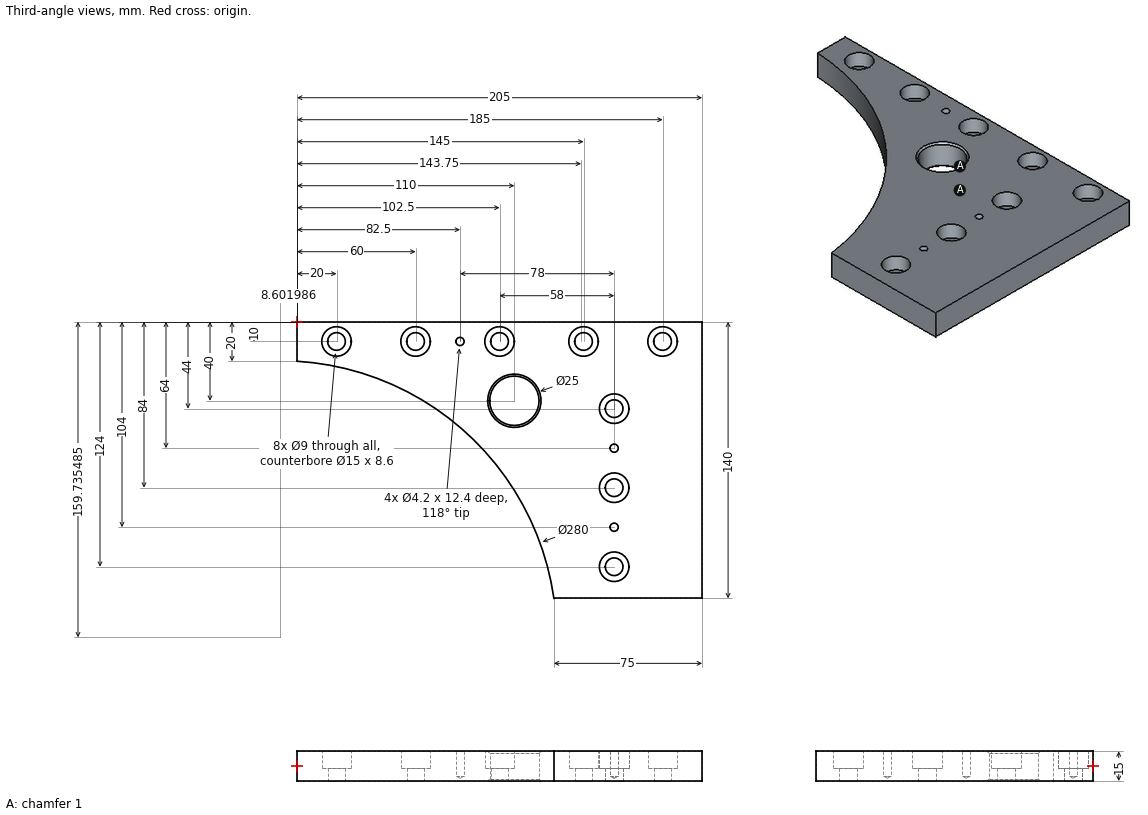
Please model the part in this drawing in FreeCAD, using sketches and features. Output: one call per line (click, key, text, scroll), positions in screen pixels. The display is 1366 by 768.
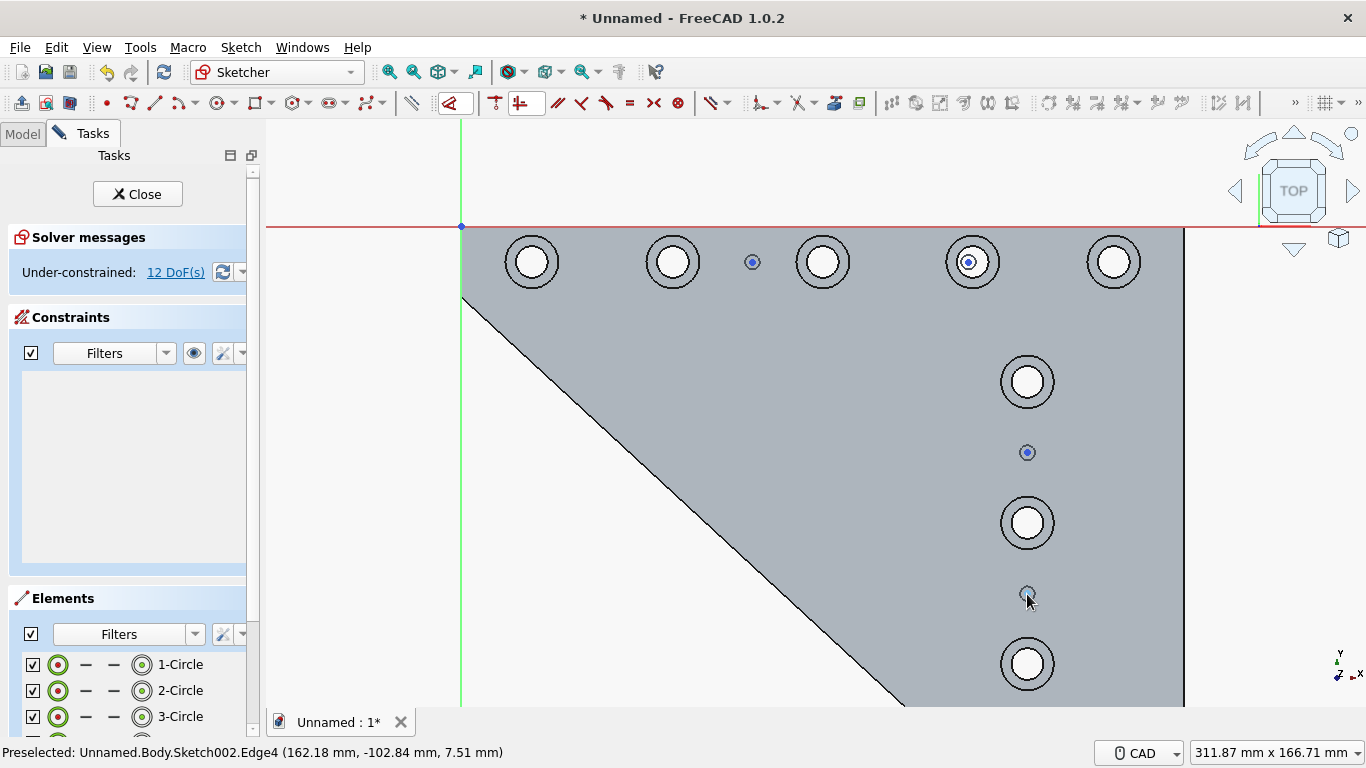
scroll(758, 257, up, 4)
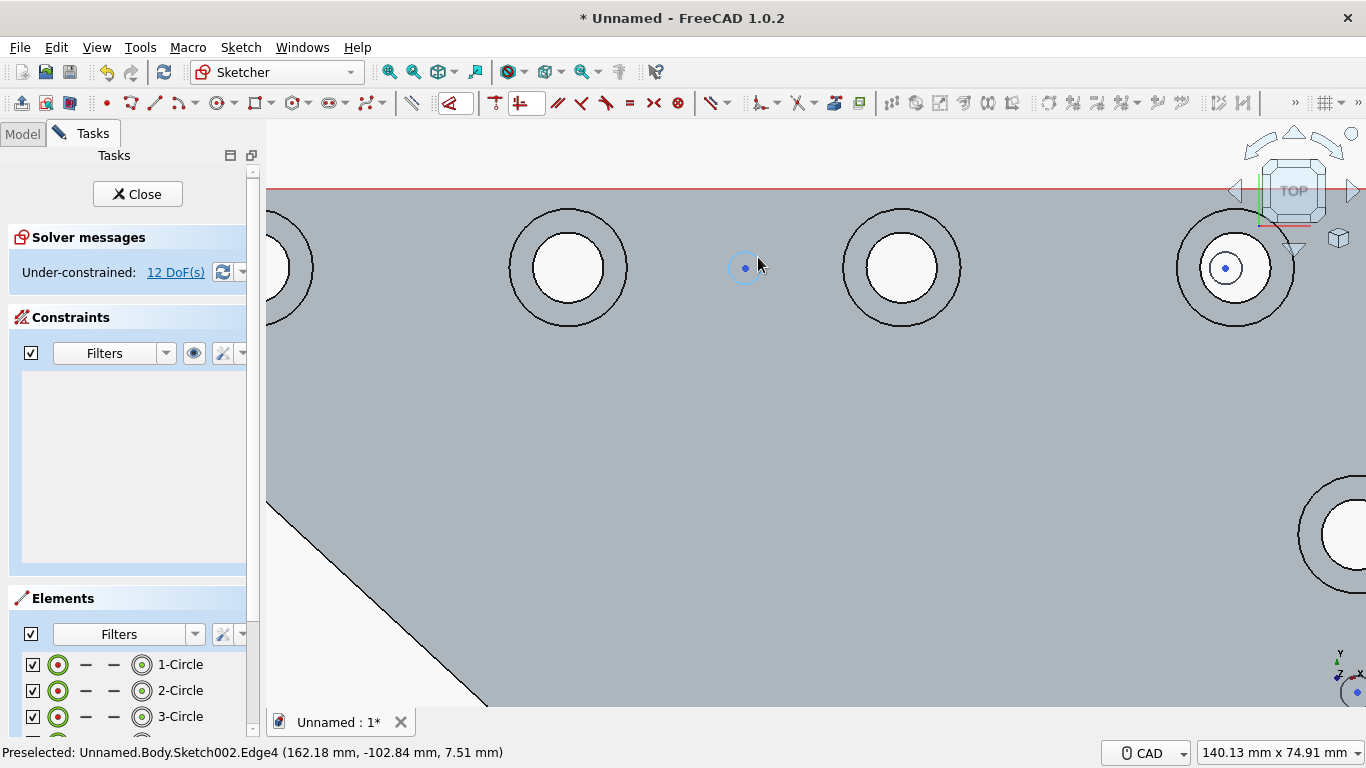
click(756, 257)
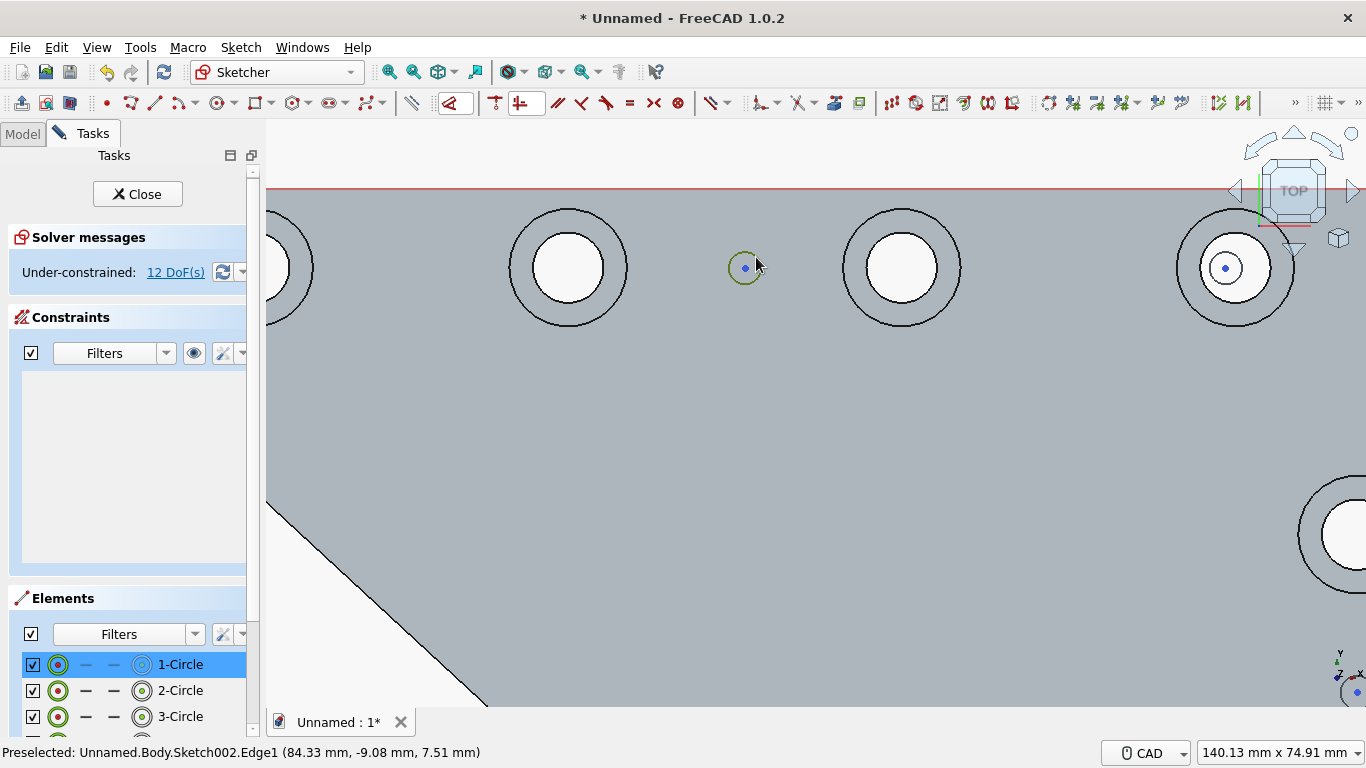
scroll(757, 256, down, 4)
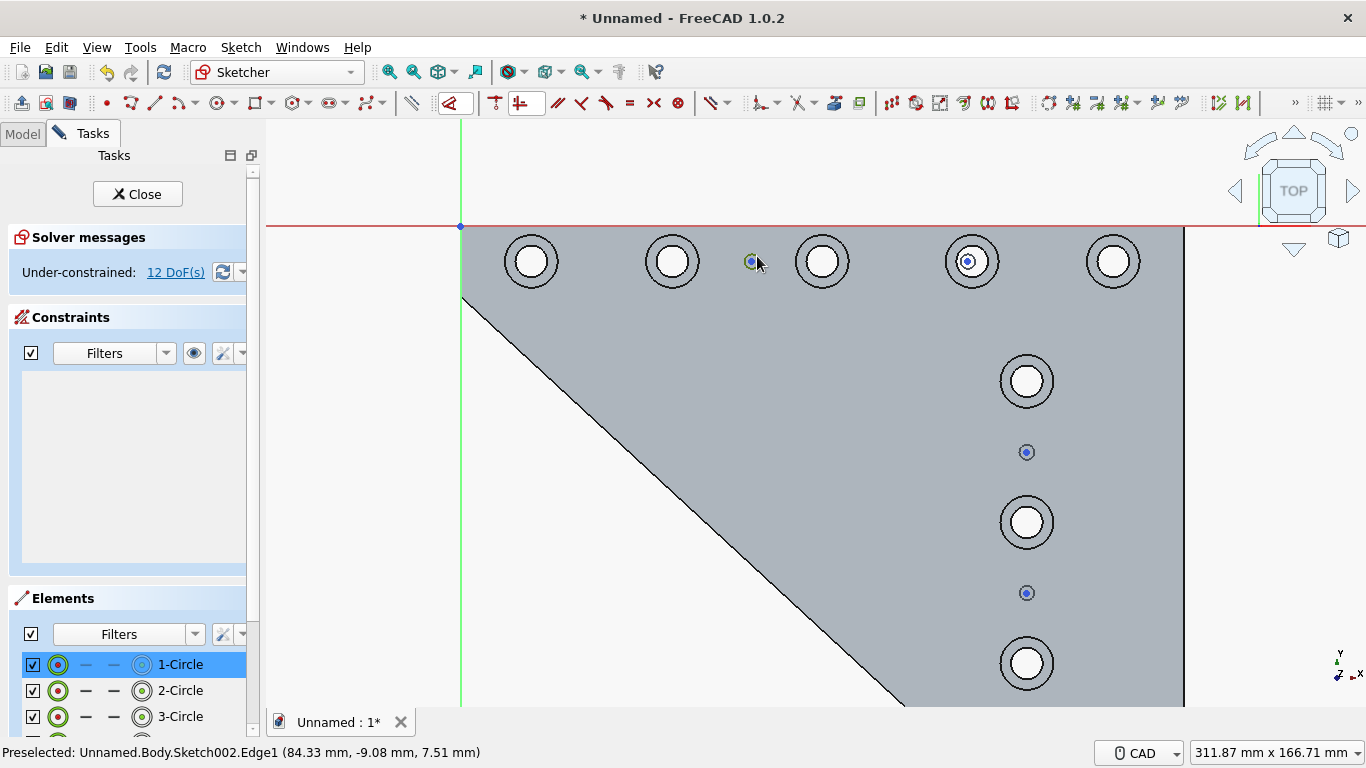
scroll(973, 256, up, 4)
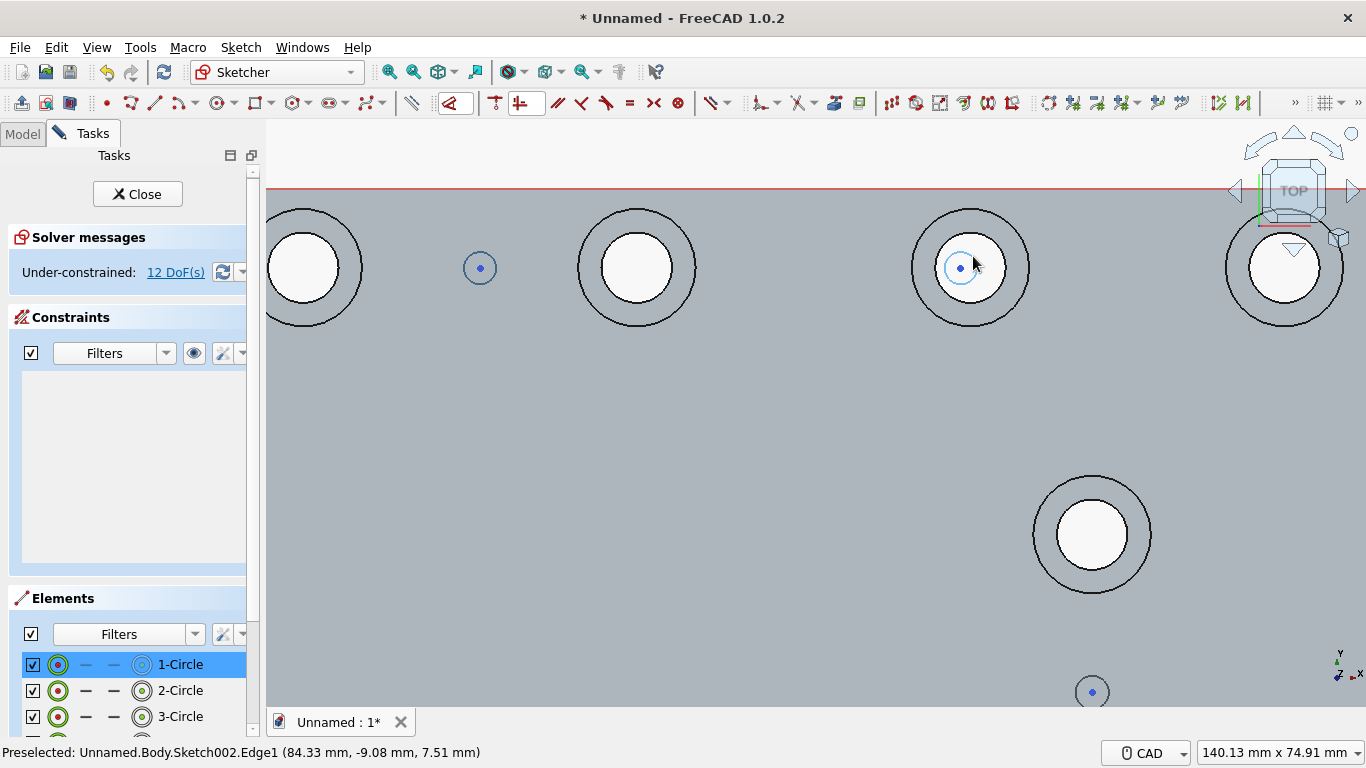
click(972, 257)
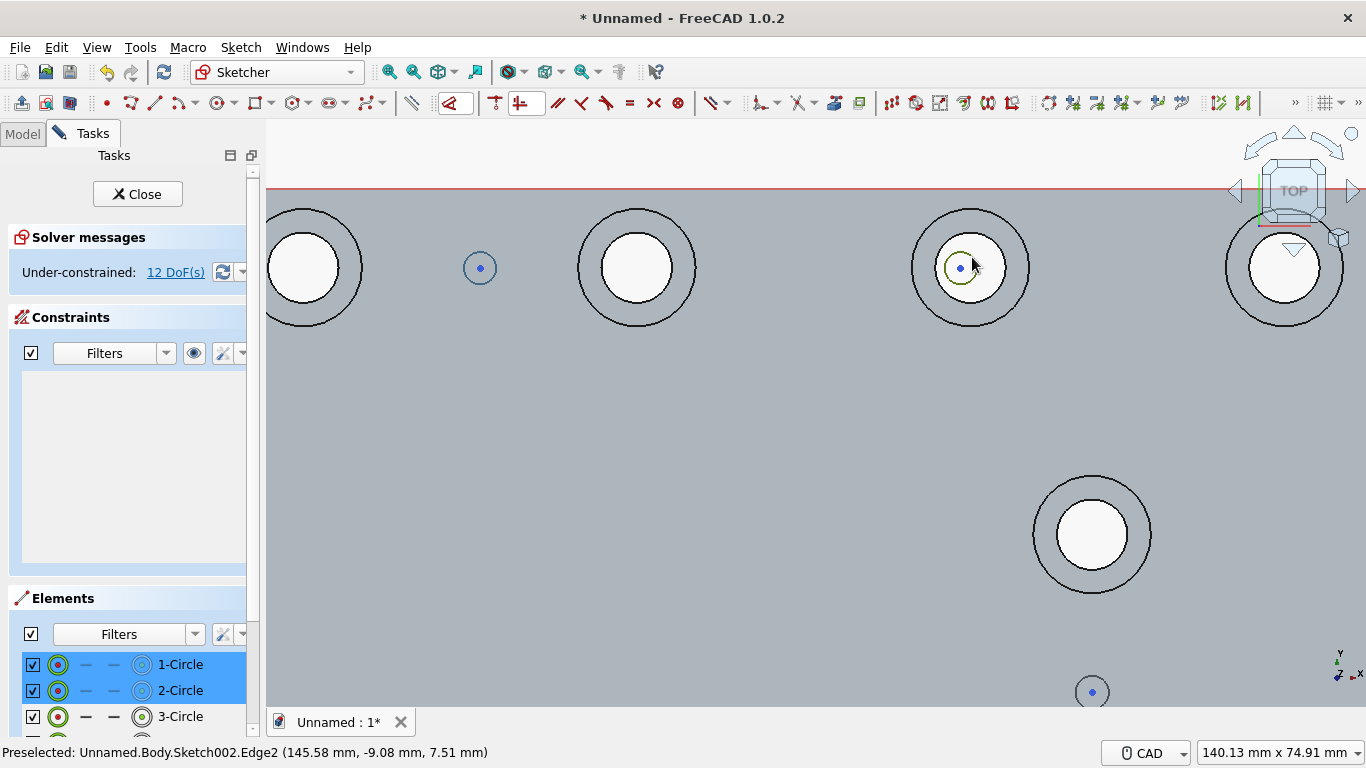
click(1093, 676)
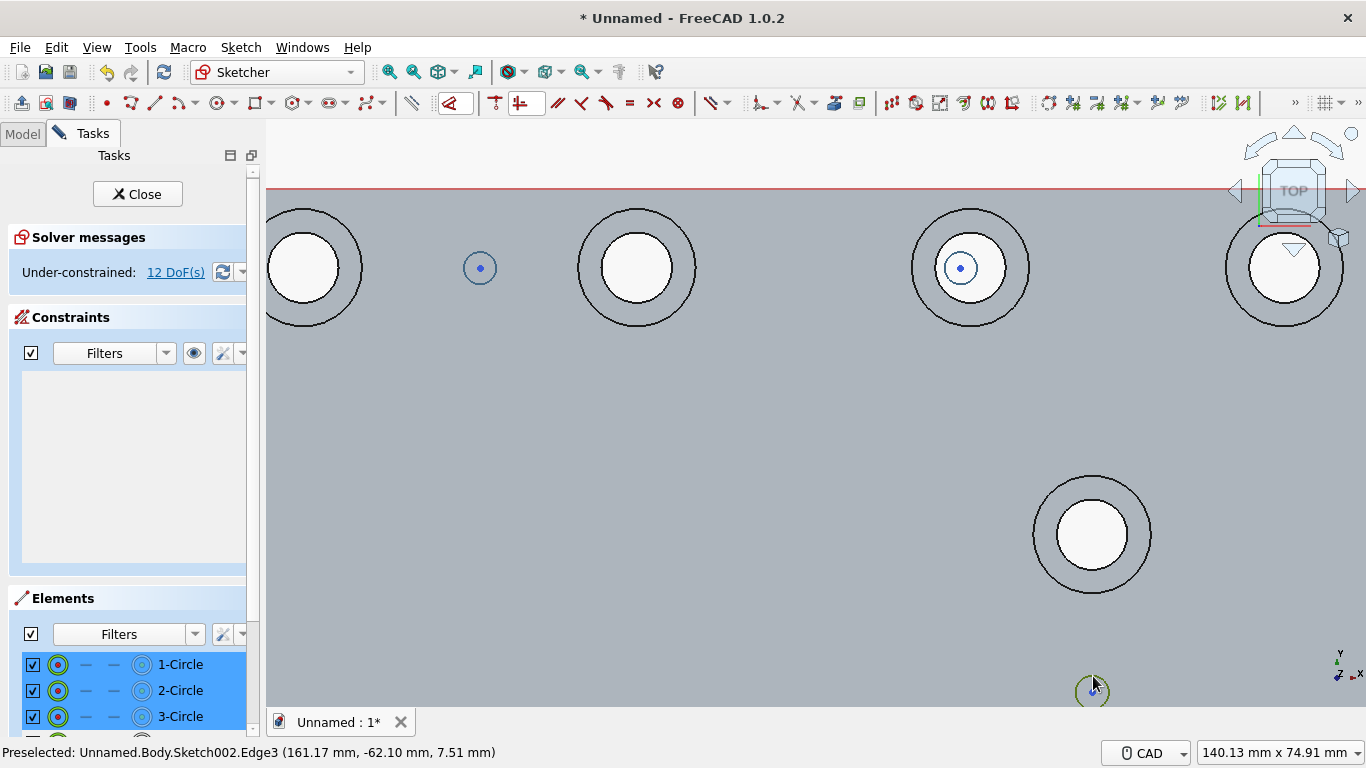
scroll(974, 256, down, 4)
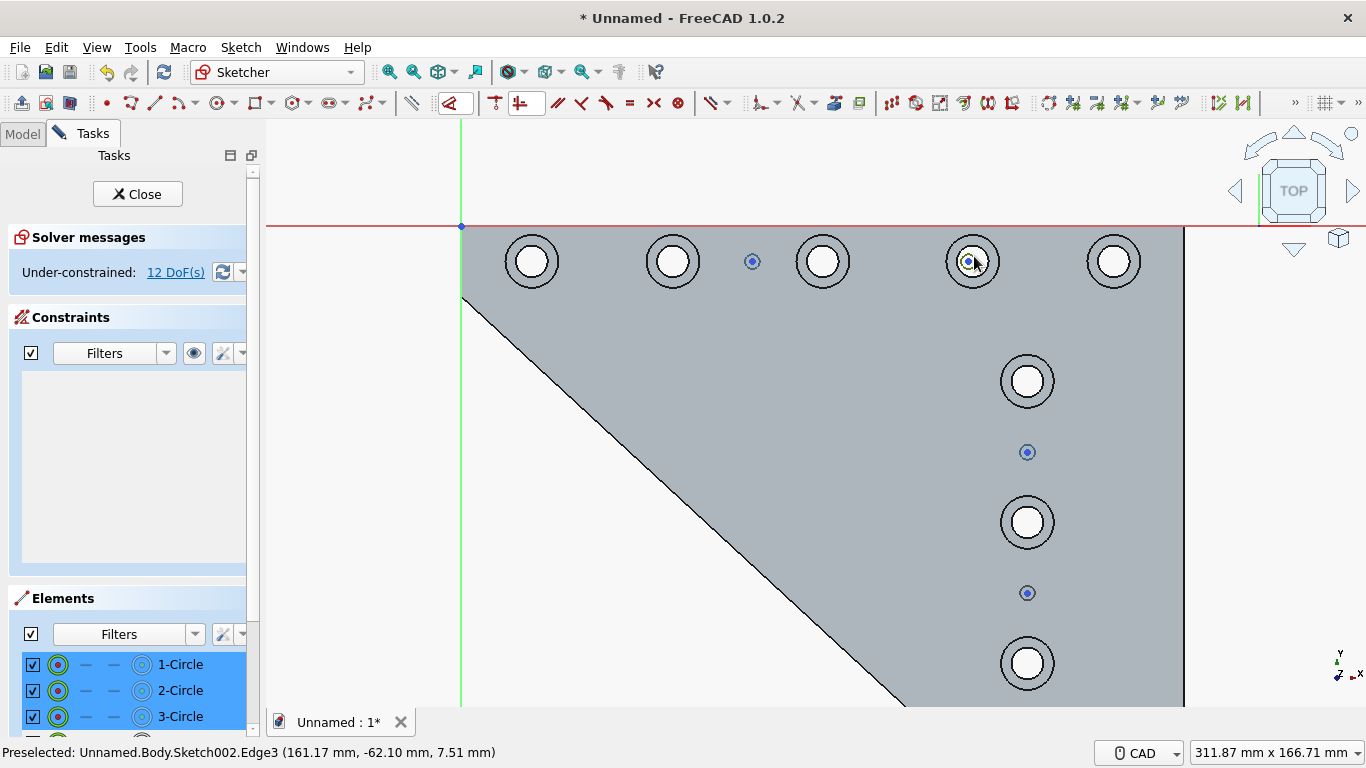
scroll(1033, 588, up, 4)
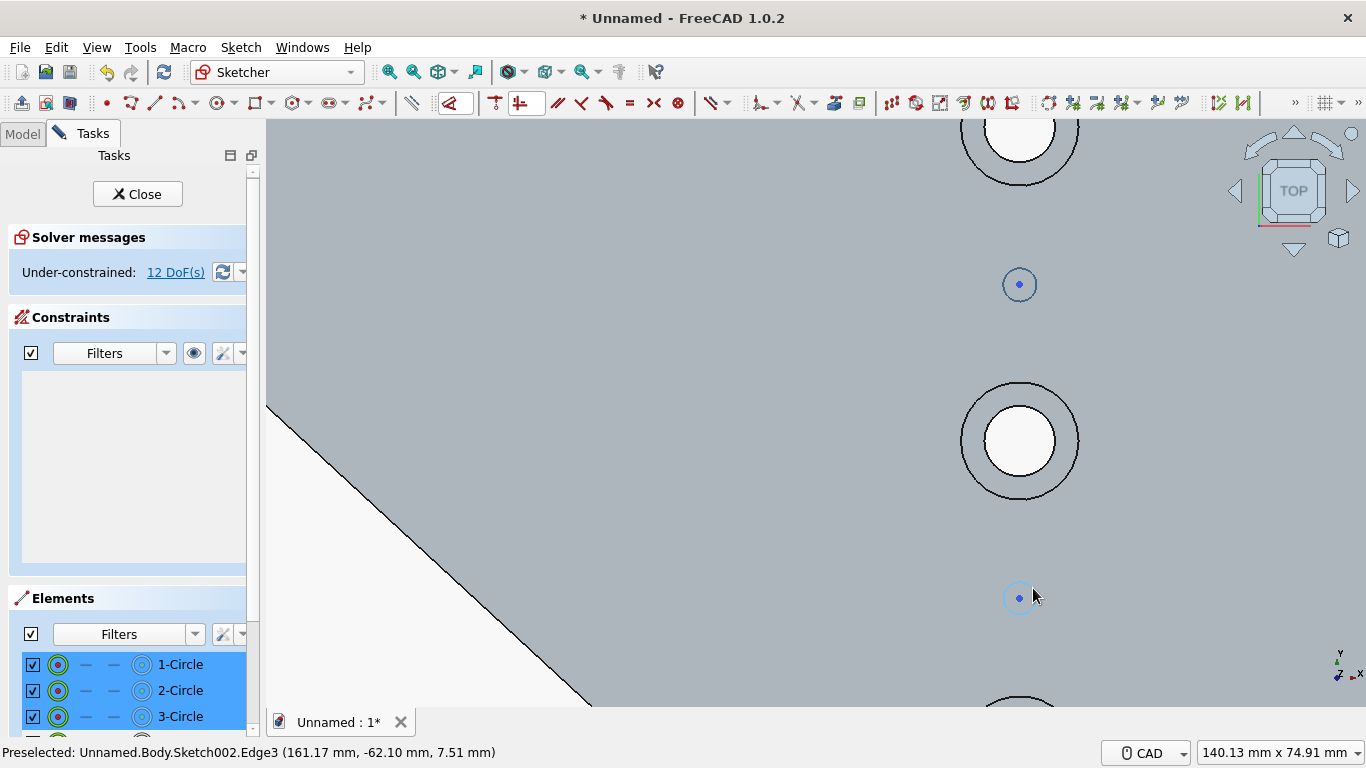
click(1031, 587)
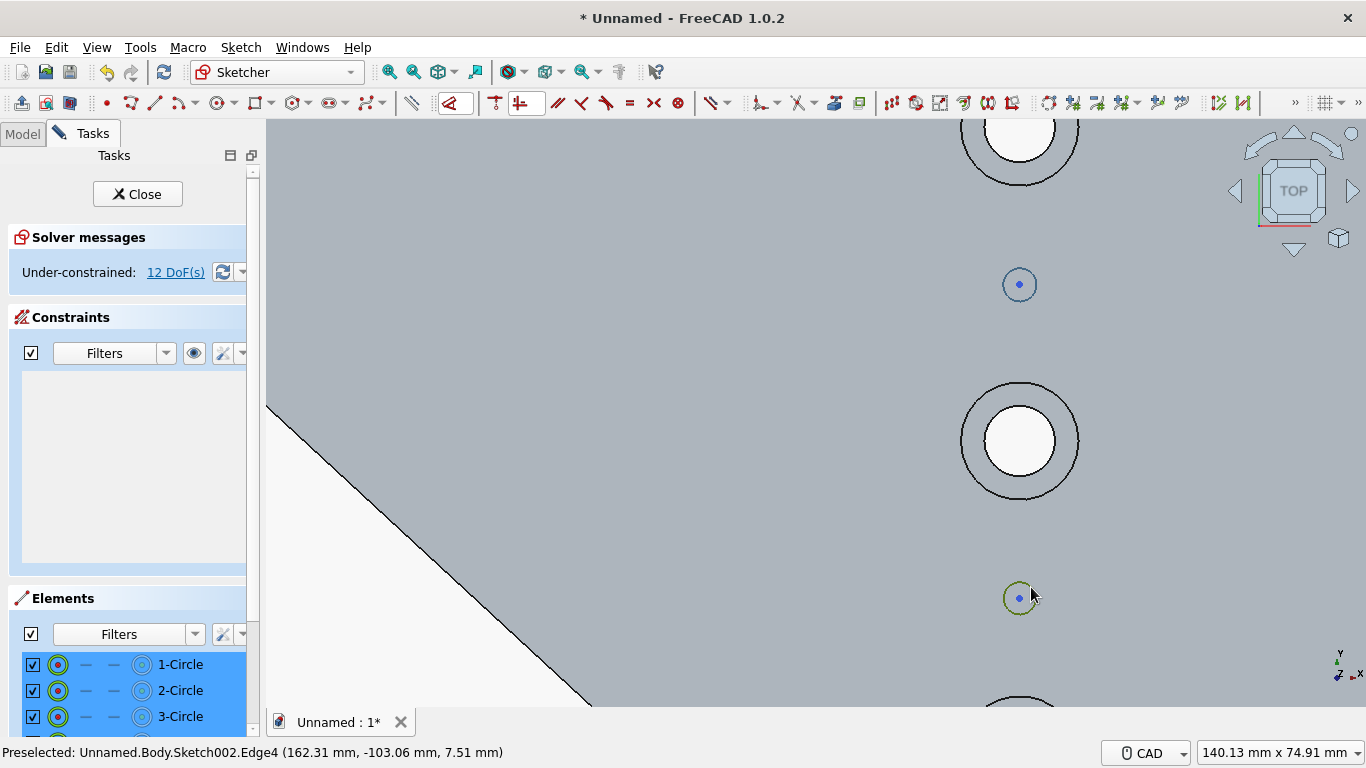
click(630, 104)